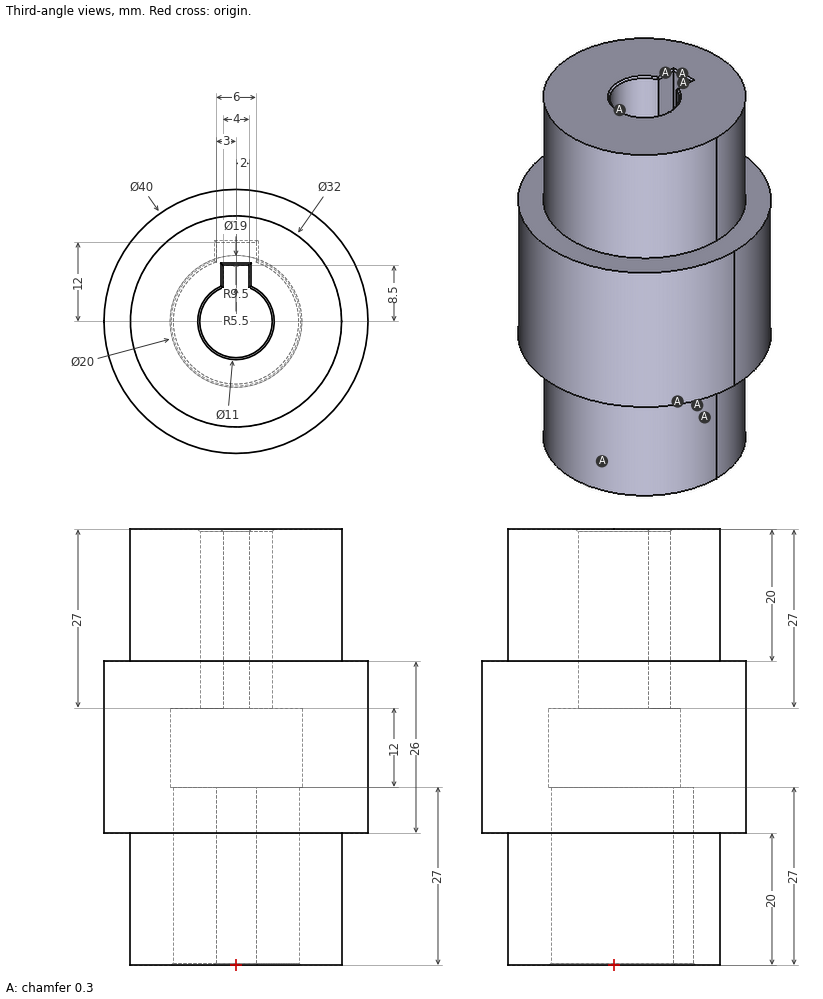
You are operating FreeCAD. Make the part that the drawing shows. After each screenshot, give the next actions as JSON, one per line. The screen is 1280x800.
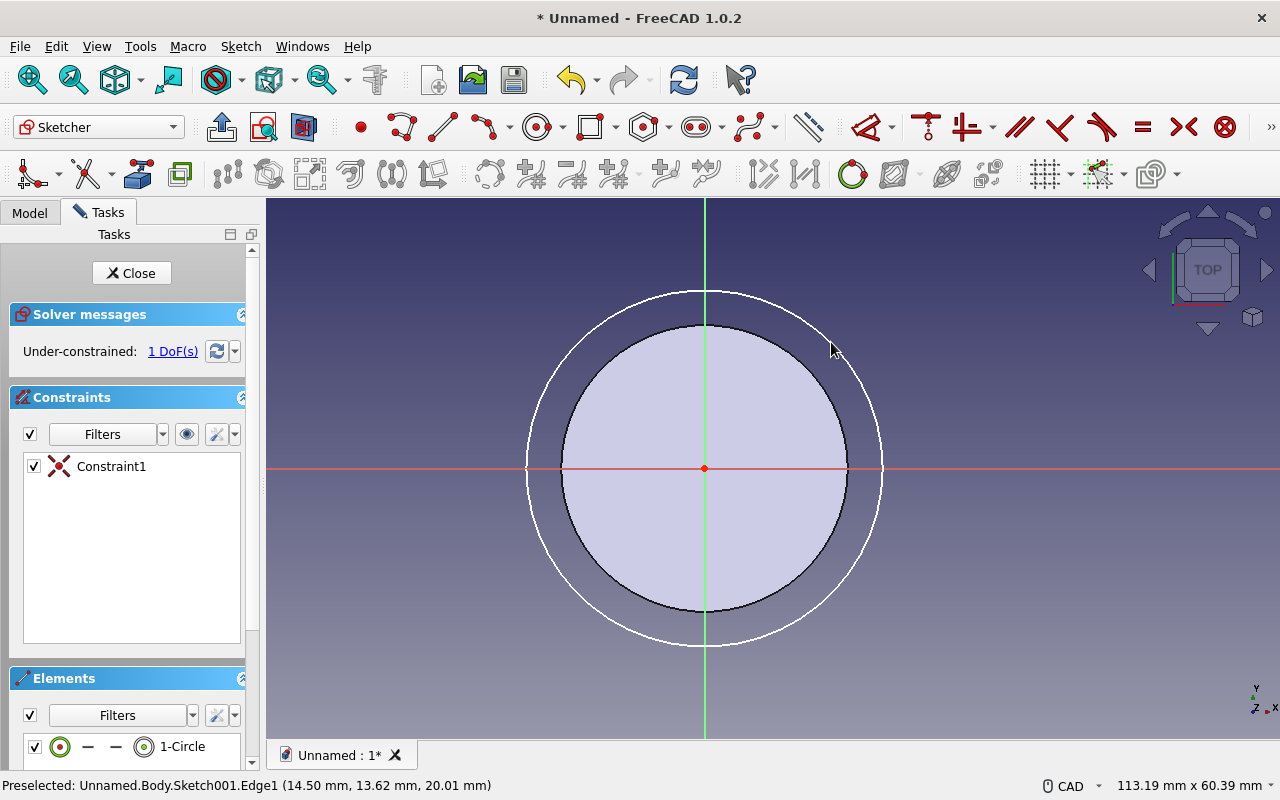
{"action": "left_click", "coordinate": [866, 128]}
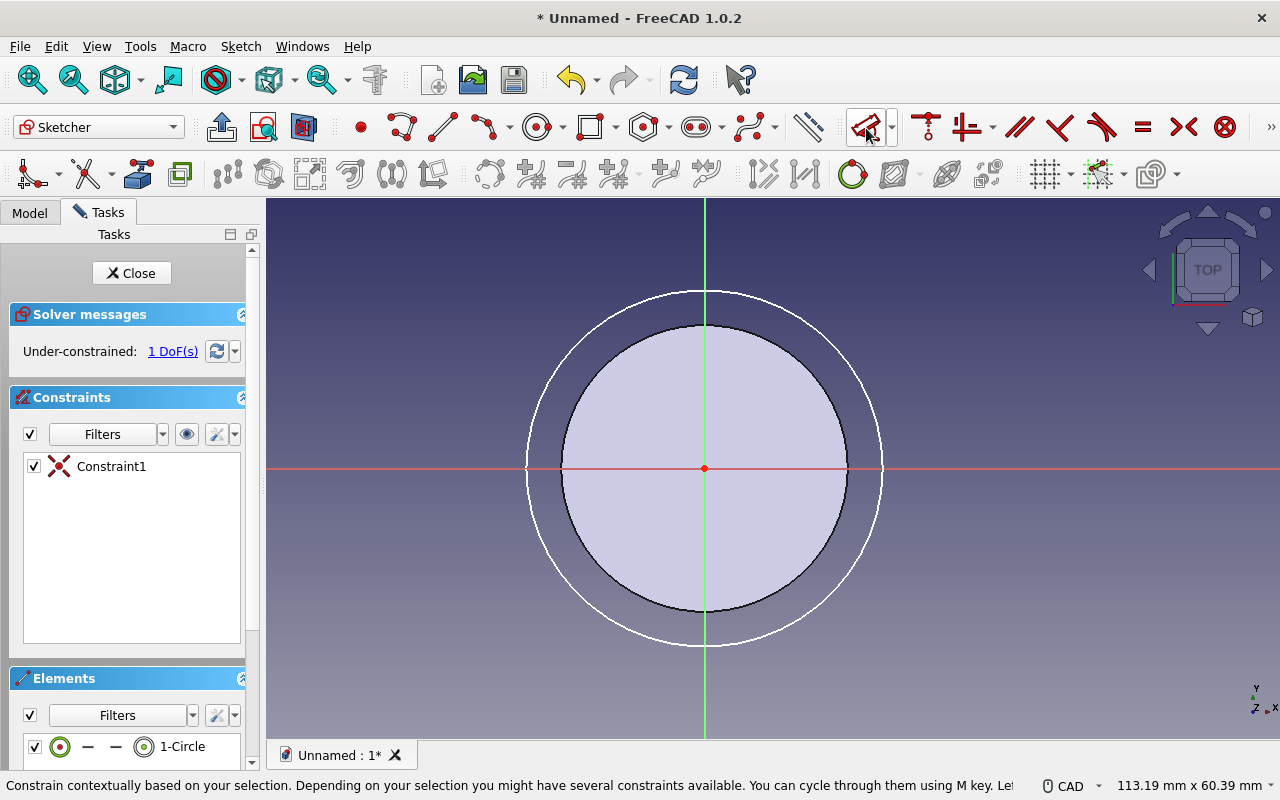
{"action": "left_click", "coordinate": [830, 342]}
{"action": "left_click", "coordinate": [853, 319]}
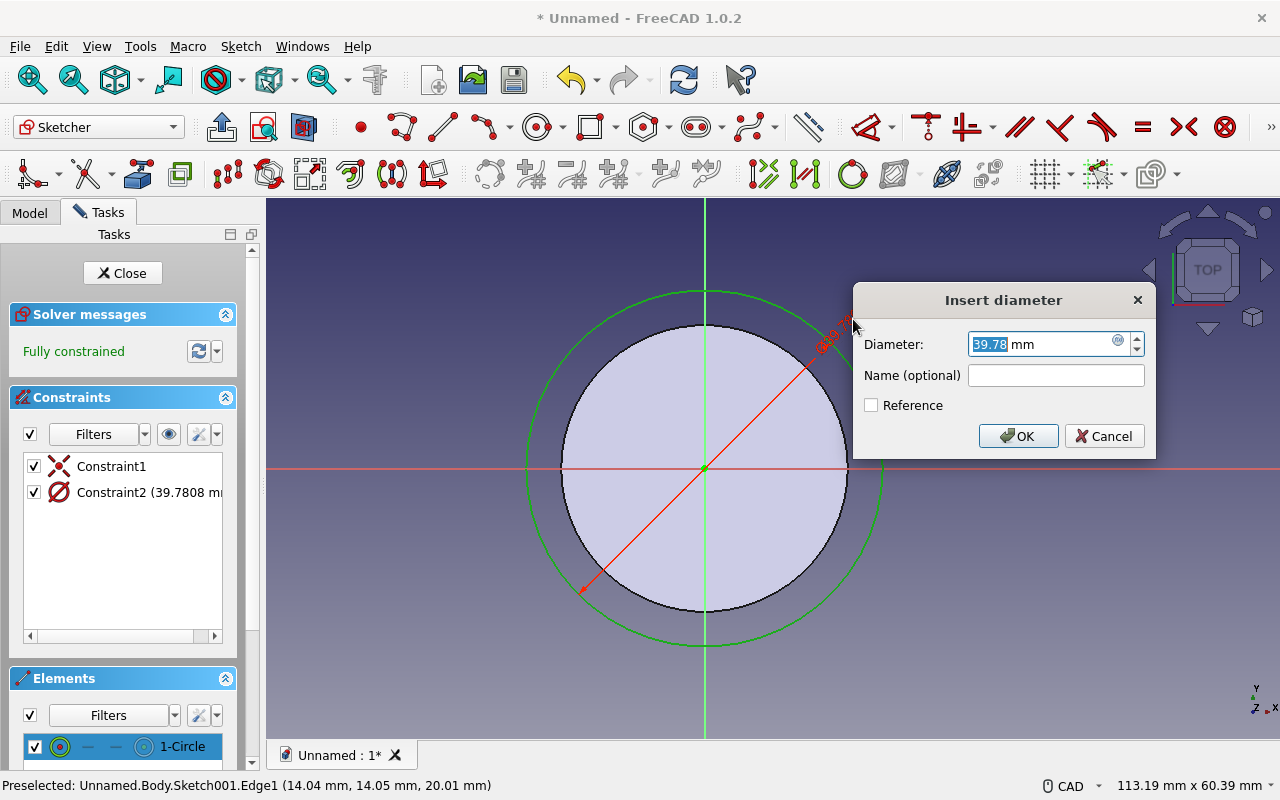
{"action": "type", "text": "40"}
{"action": "key", "text": "Return"}
{"action": "key", "text": "Escape"}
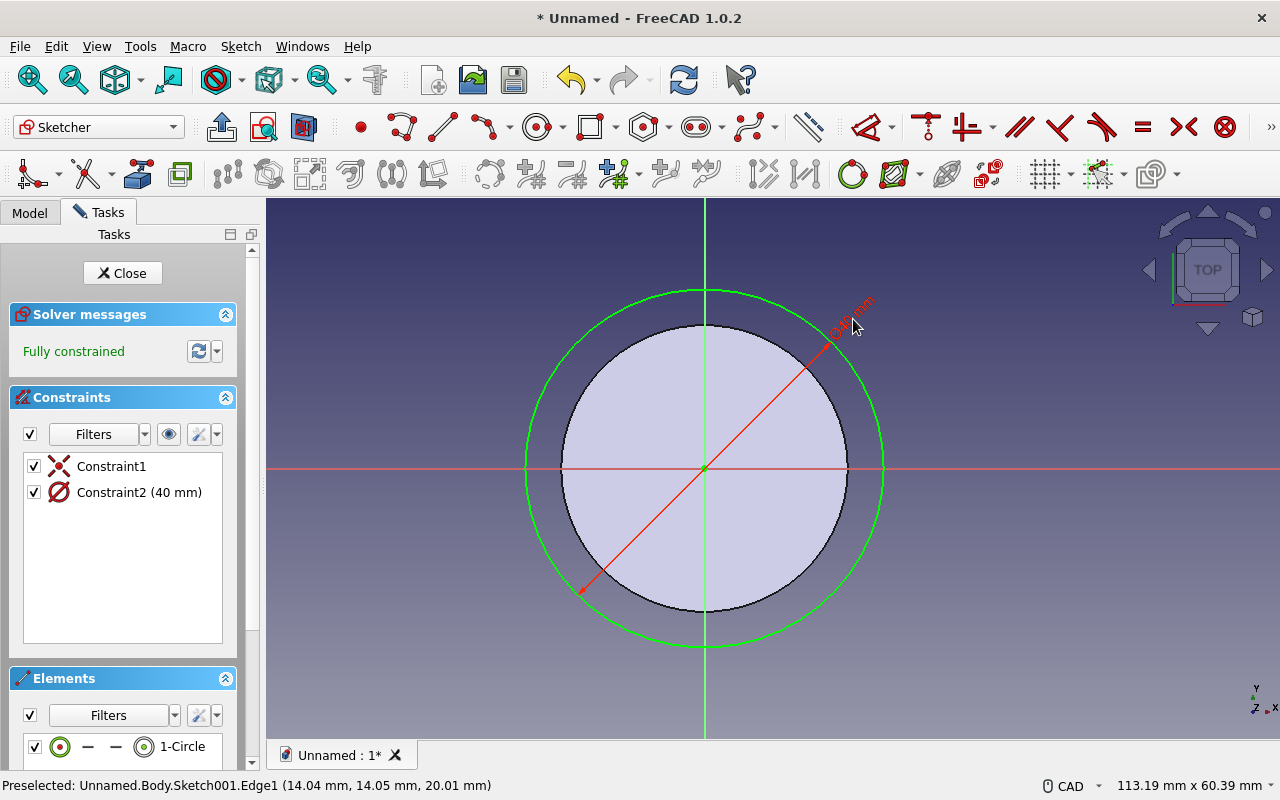
{"action": "left_click", "coordinate": [123, 273]}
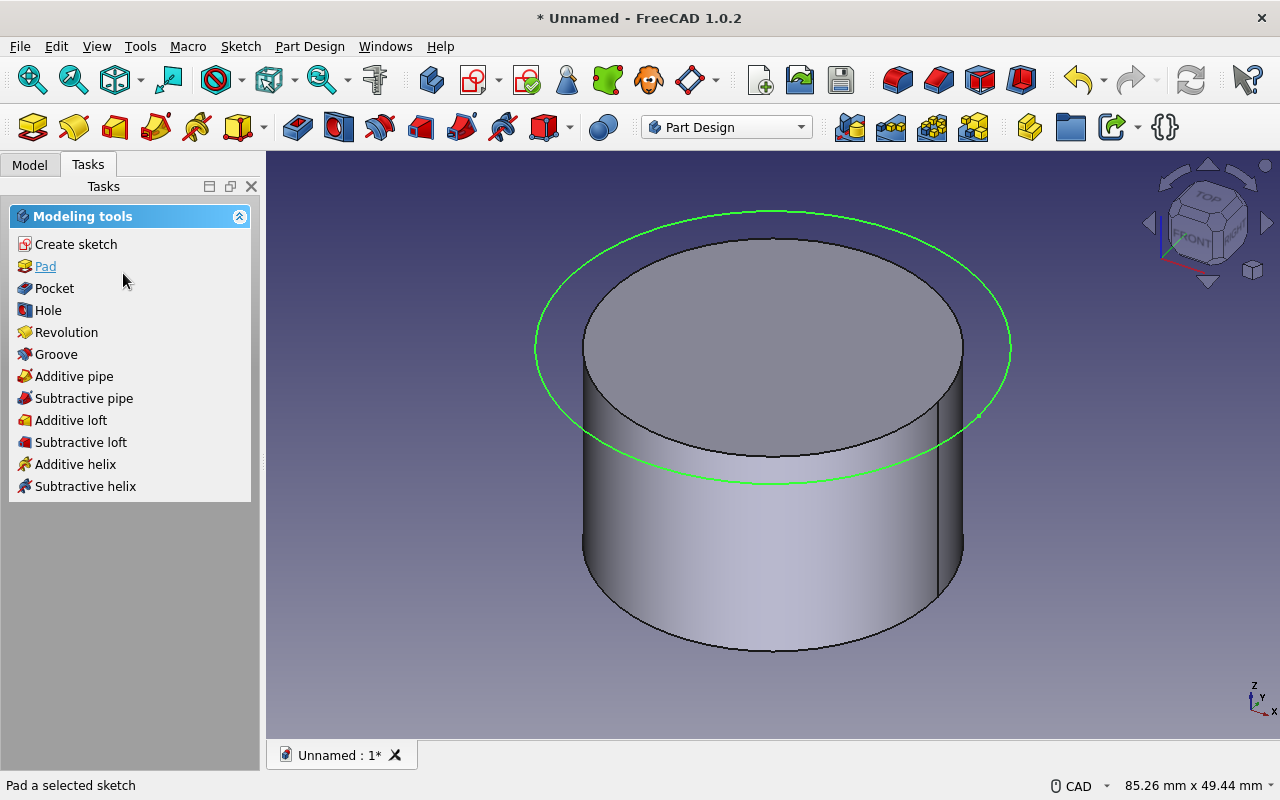
{"action": "left_click", "coordinate": [33, 128]}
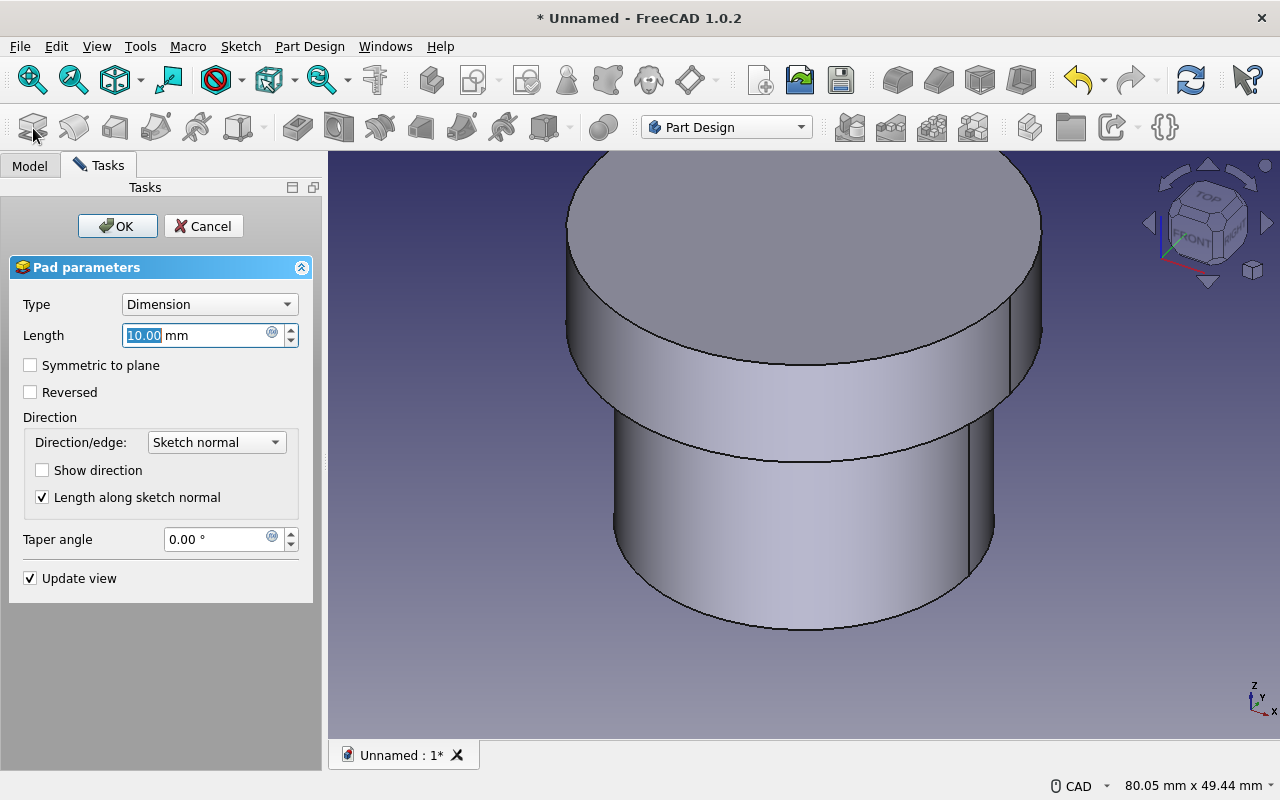
{"action": "type", "text": "26"}
{"action": "key", "text": "Tab"}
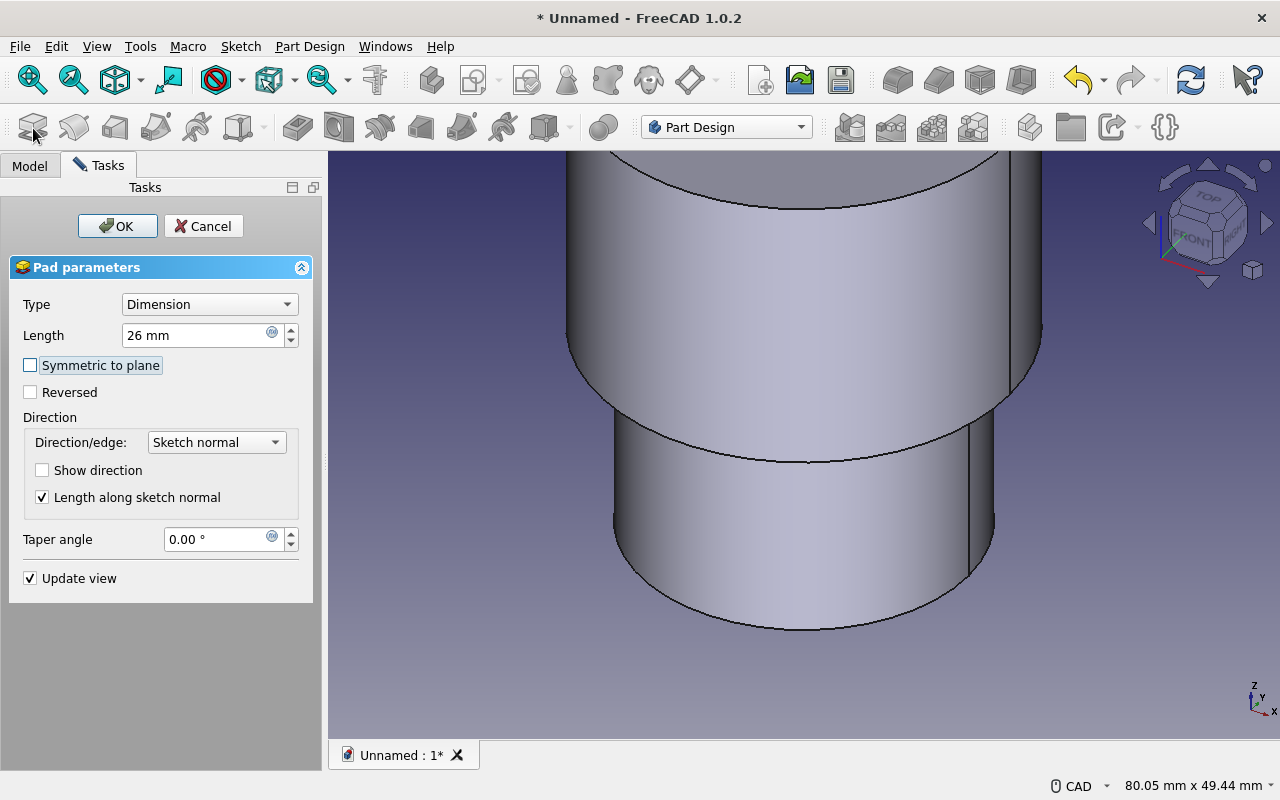
{"action": "left_click", "coordinate": [118, 226]}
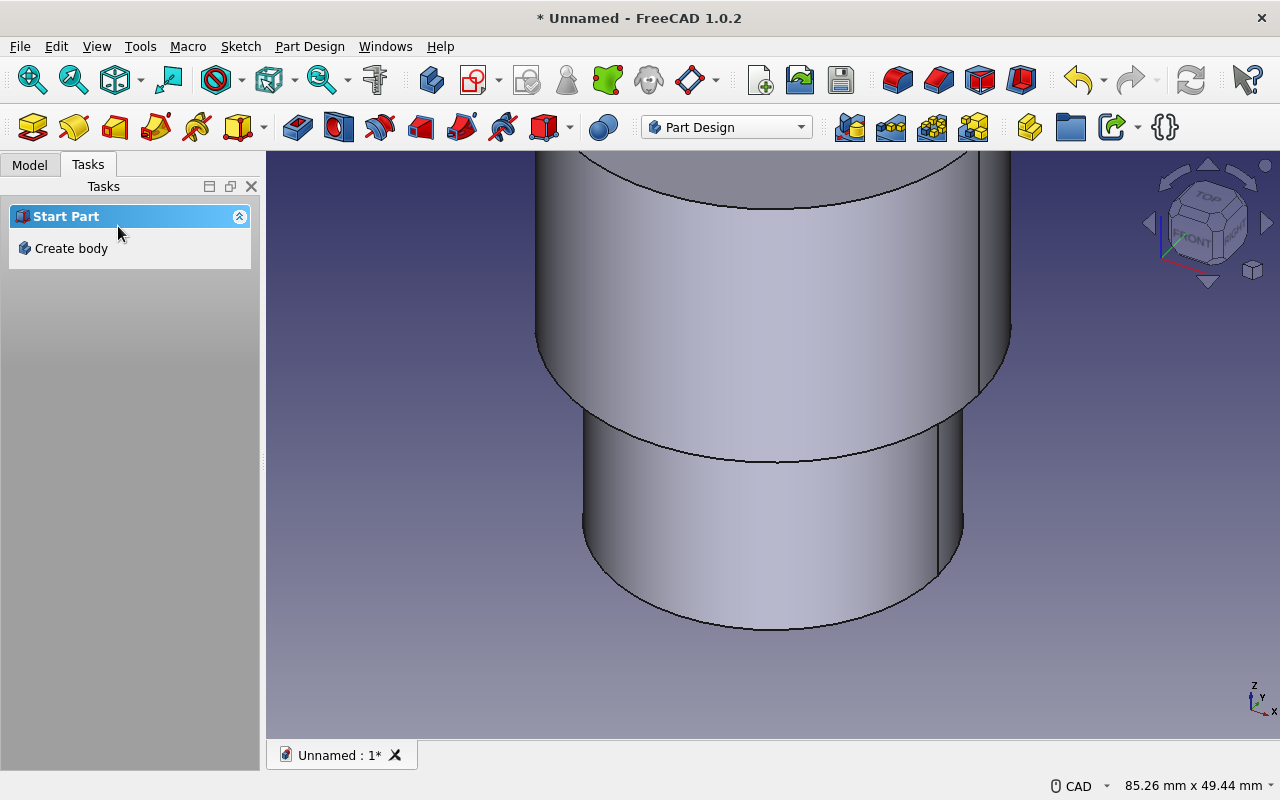
{"action": "left_click", "coordinate": [33, 80]}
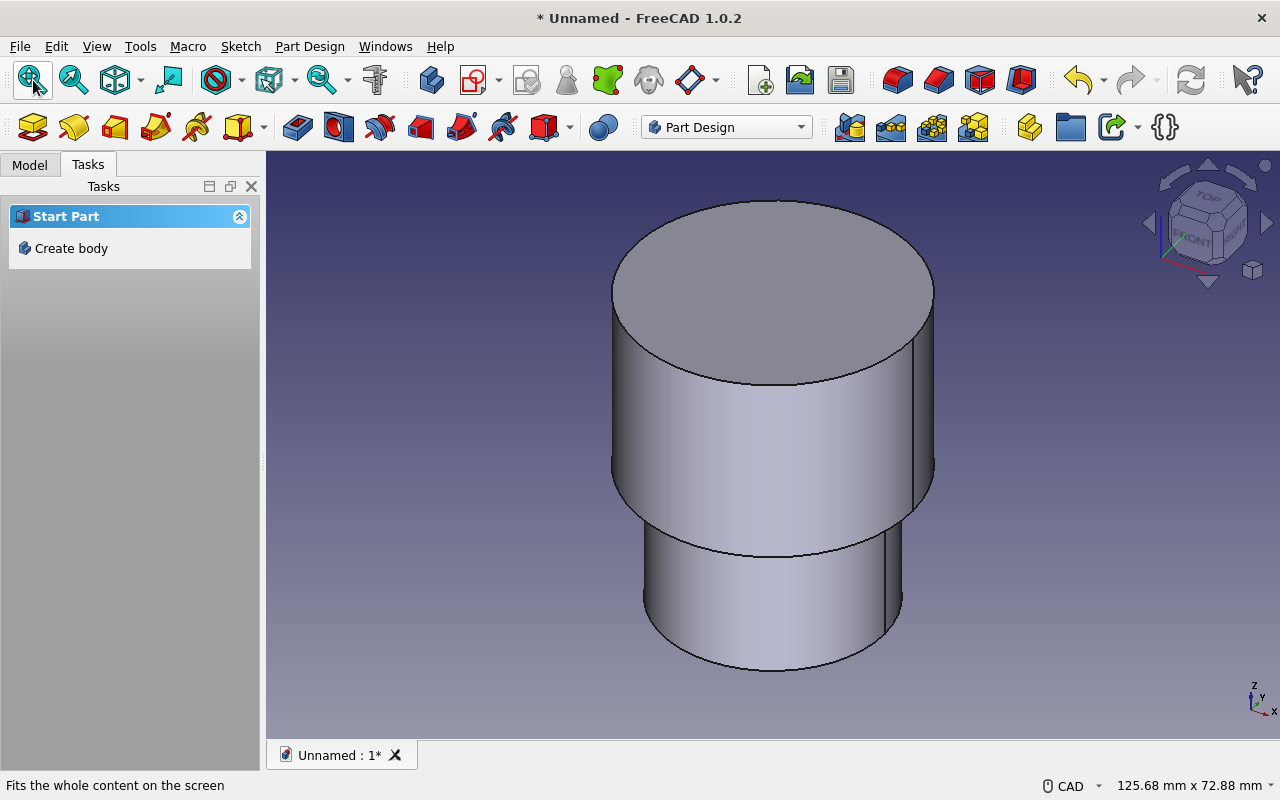
{"action": "left_click", "coordinate": [773, 292]}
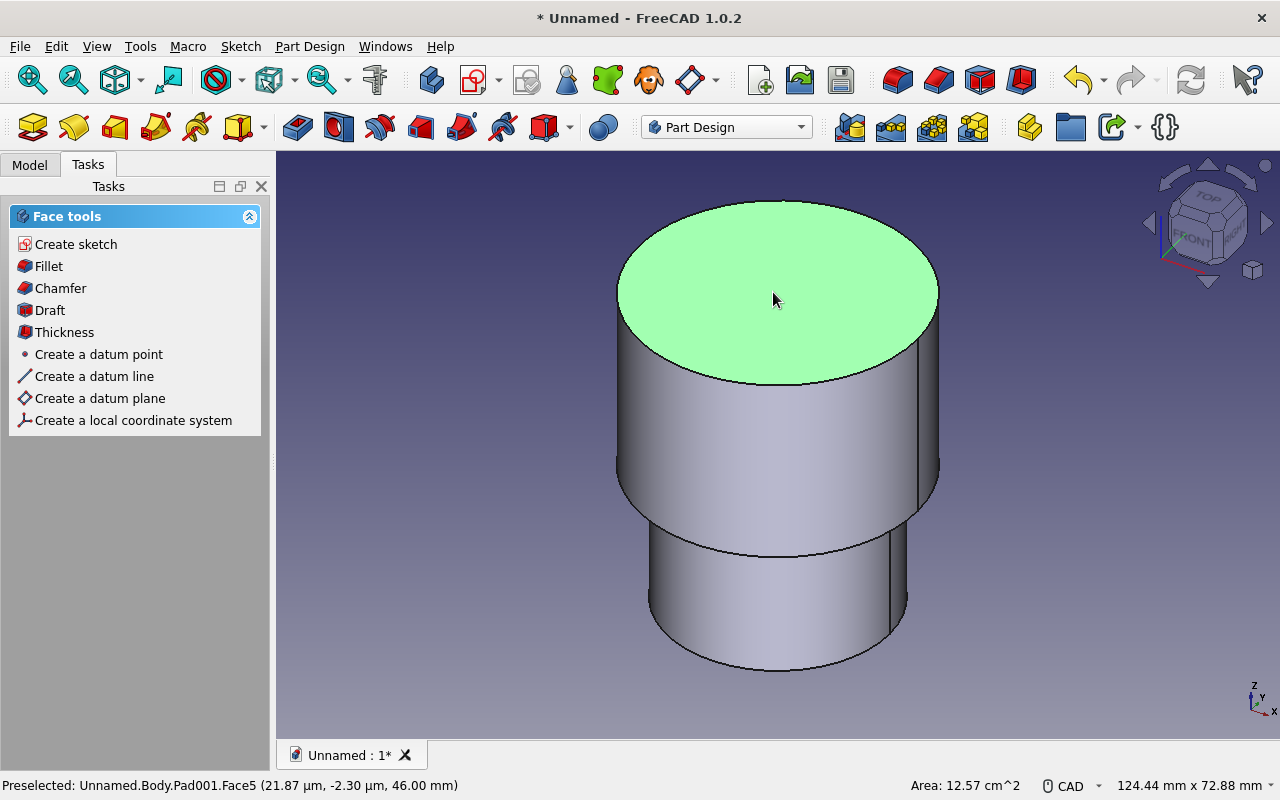
{"action": "left_click", "coordinate": [472, 80]}